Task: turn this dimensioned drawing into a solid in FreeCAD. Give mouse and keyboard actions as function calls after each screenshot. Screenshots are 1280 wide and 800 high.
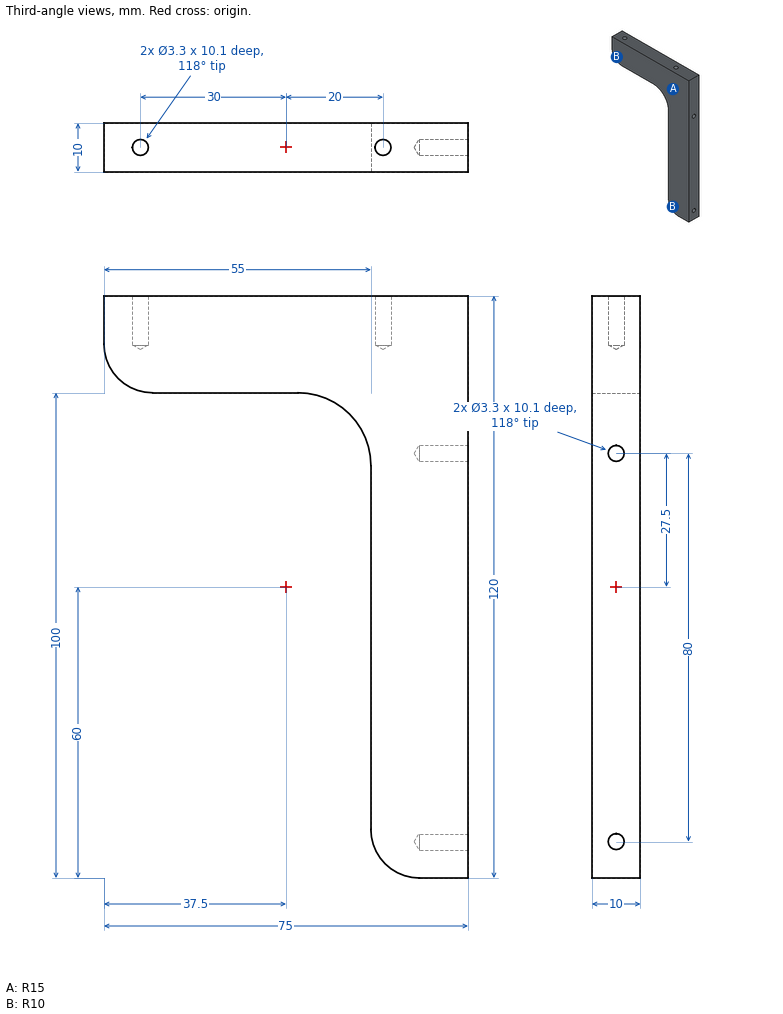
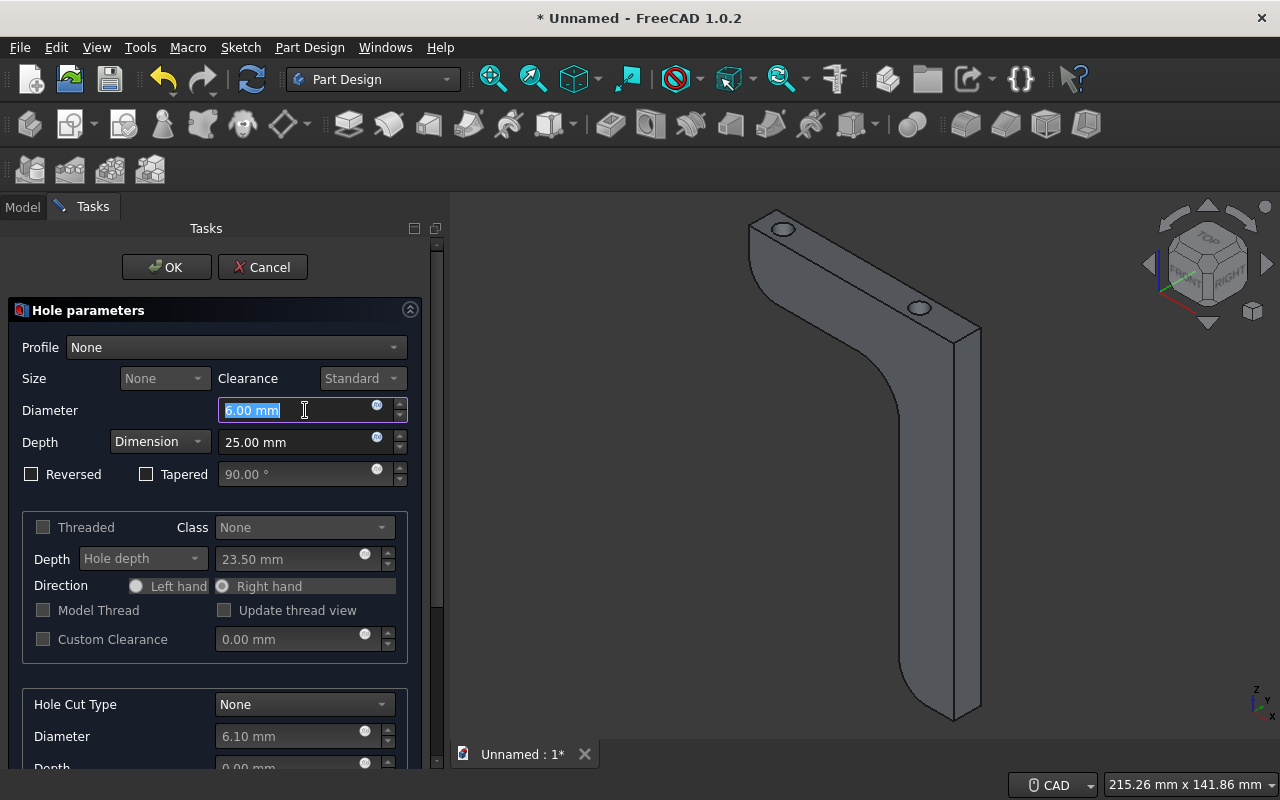
text(3.3)
key(Tab)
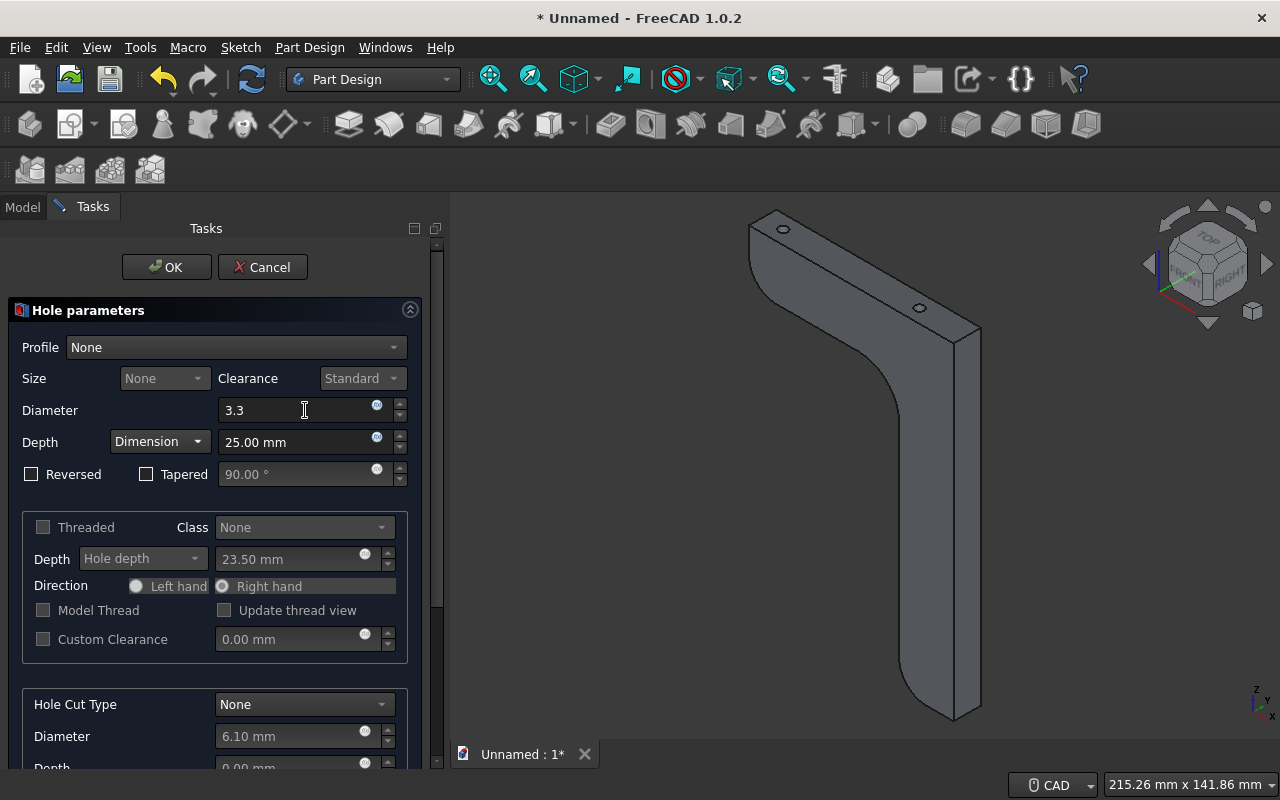
triple_click(305, 442)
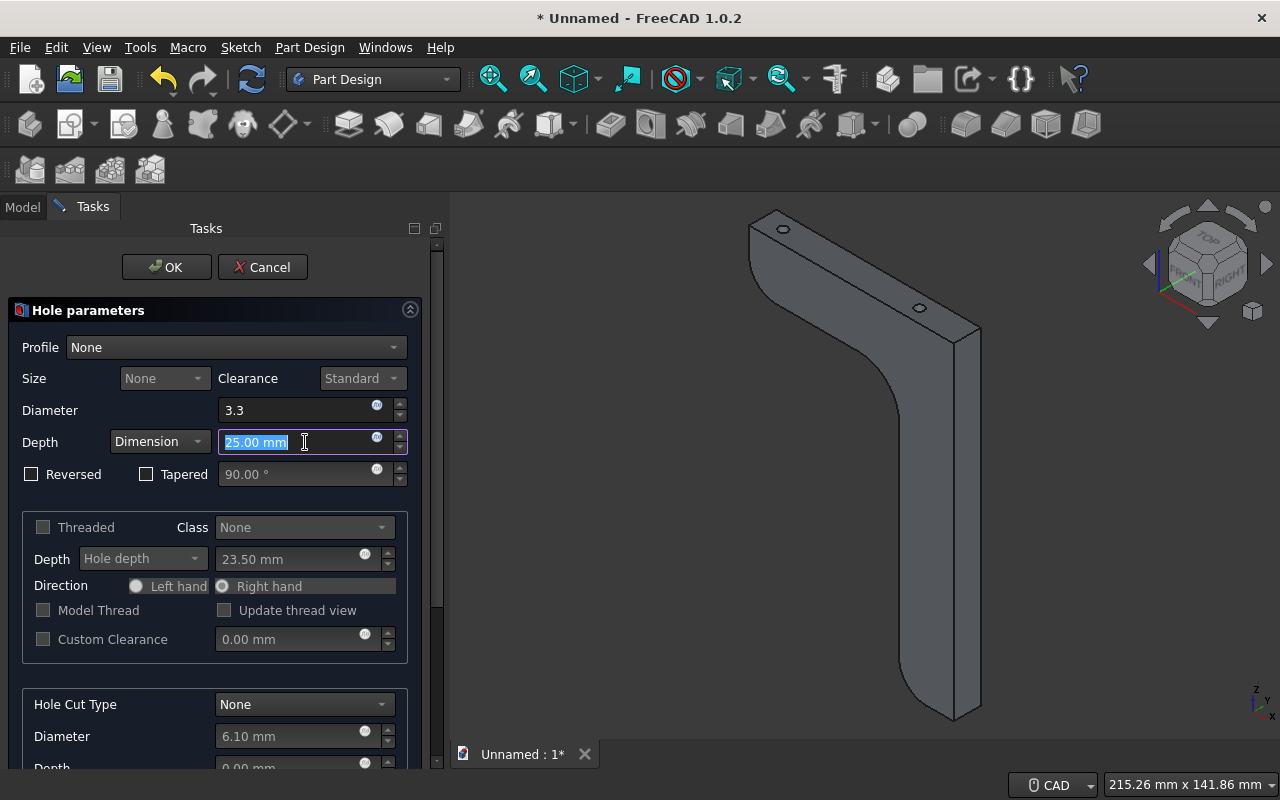
text(10.1)
key(Tab)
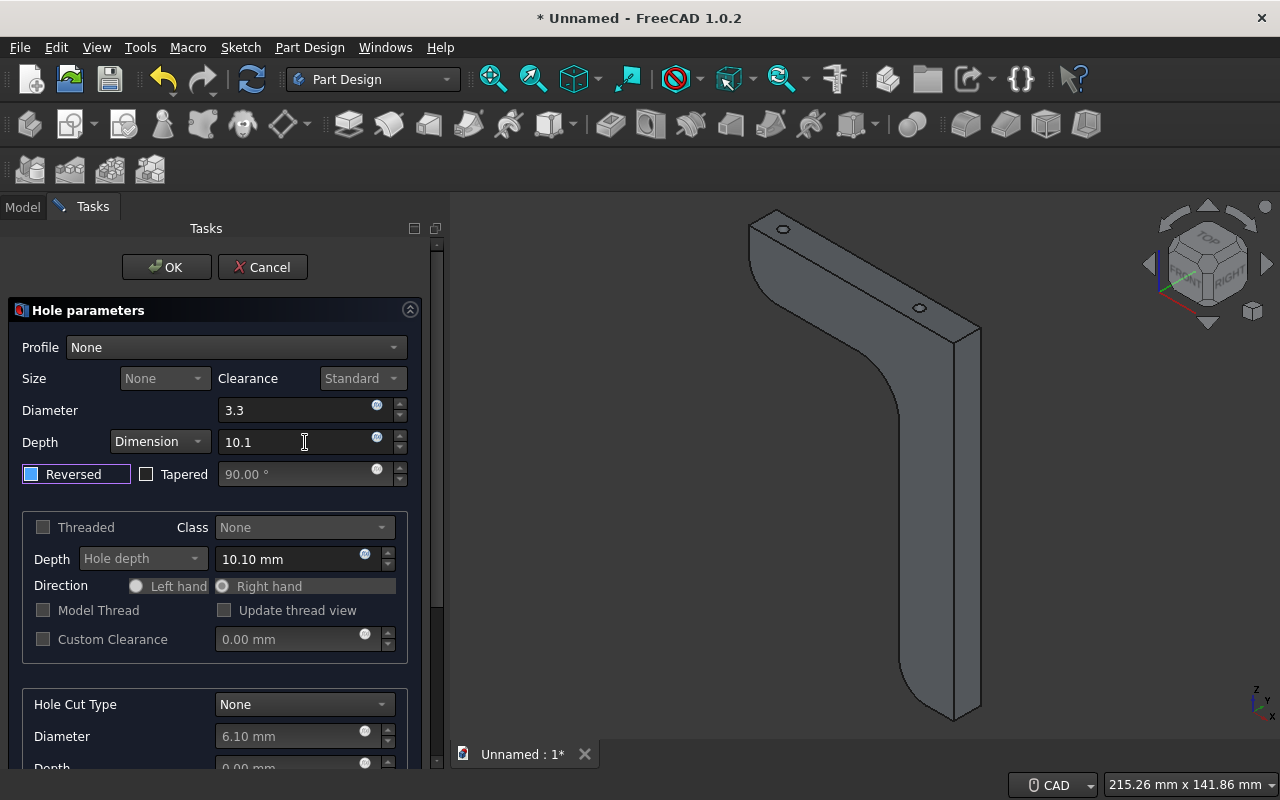
click(167, 267)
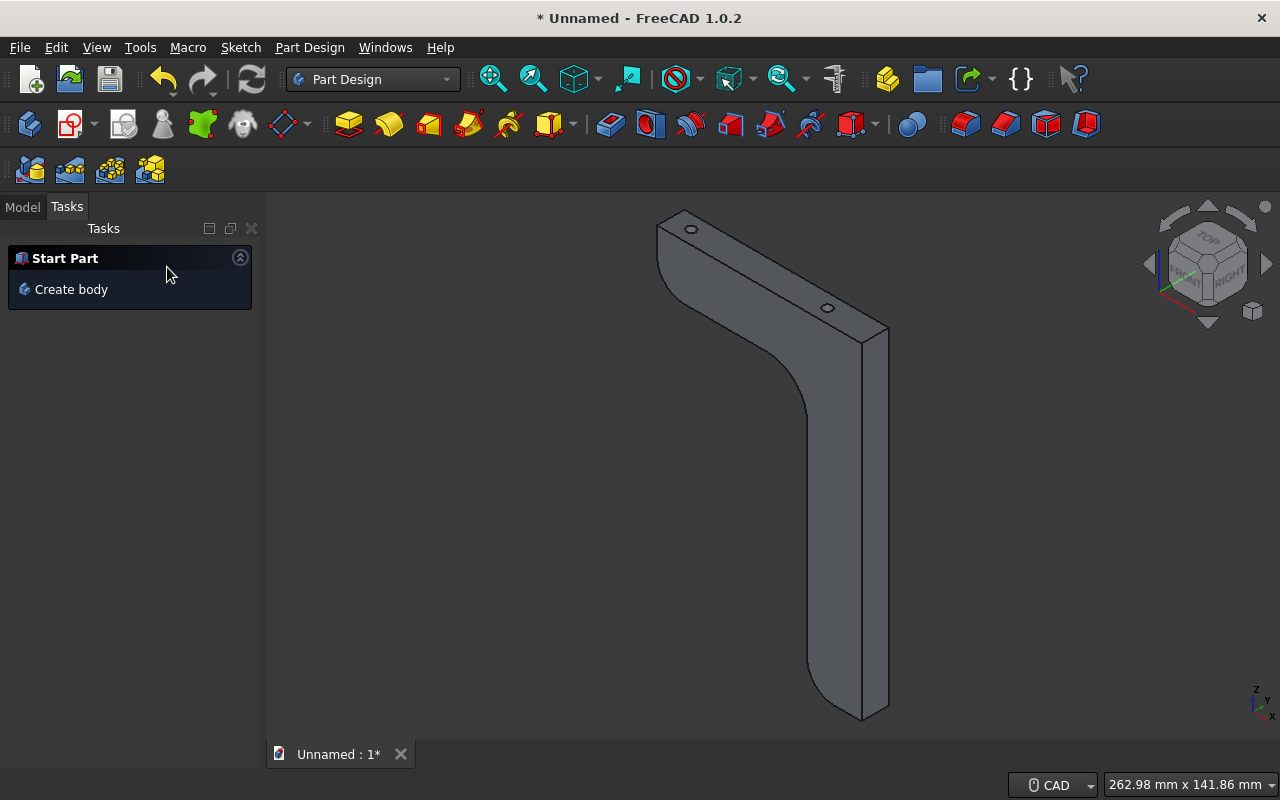
click(875, 362)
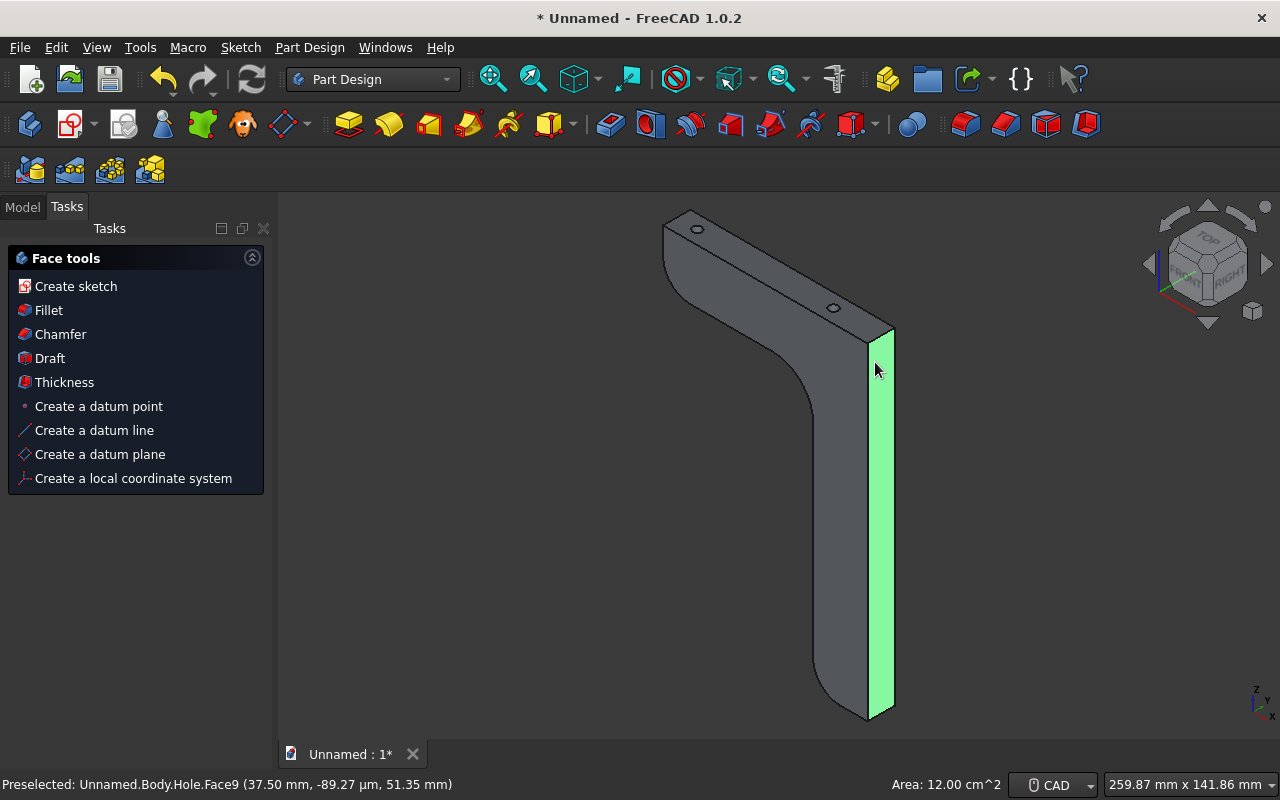
click(70, 124)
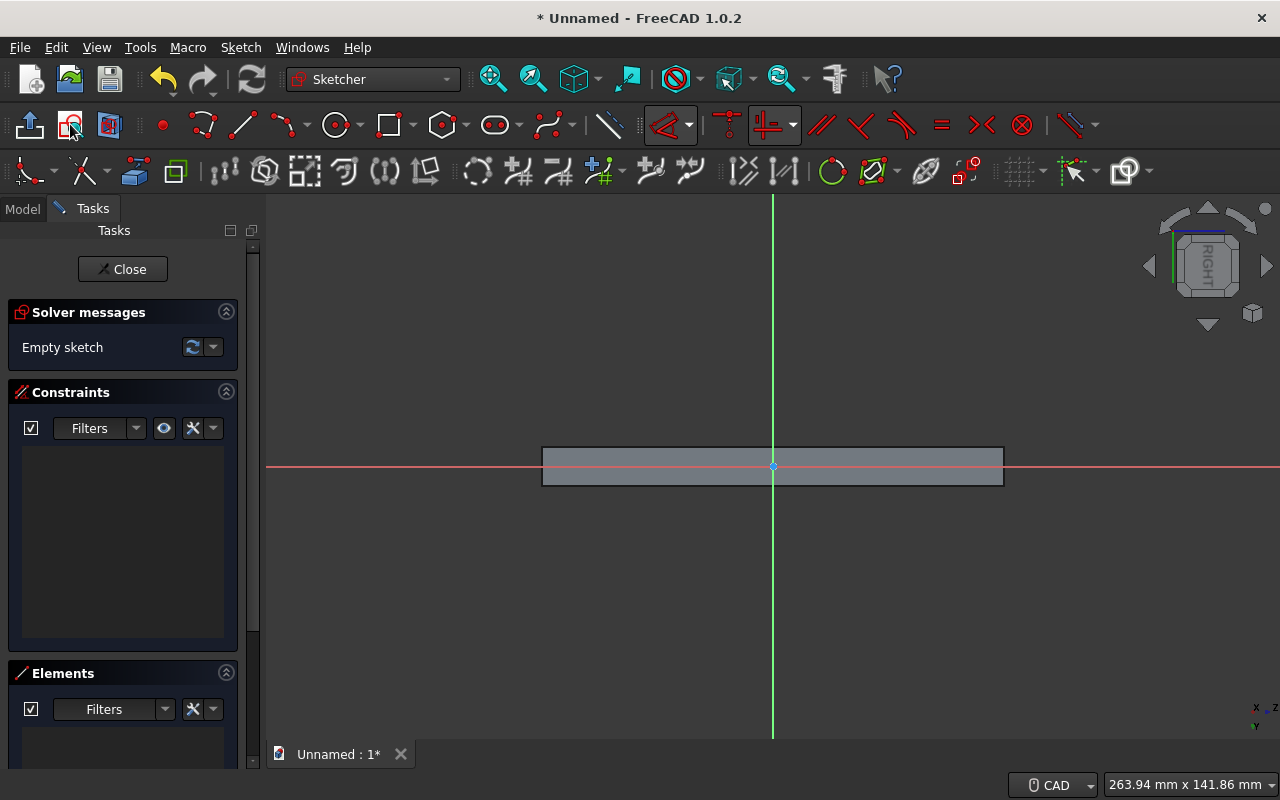
scroll(750, 467, up, 3)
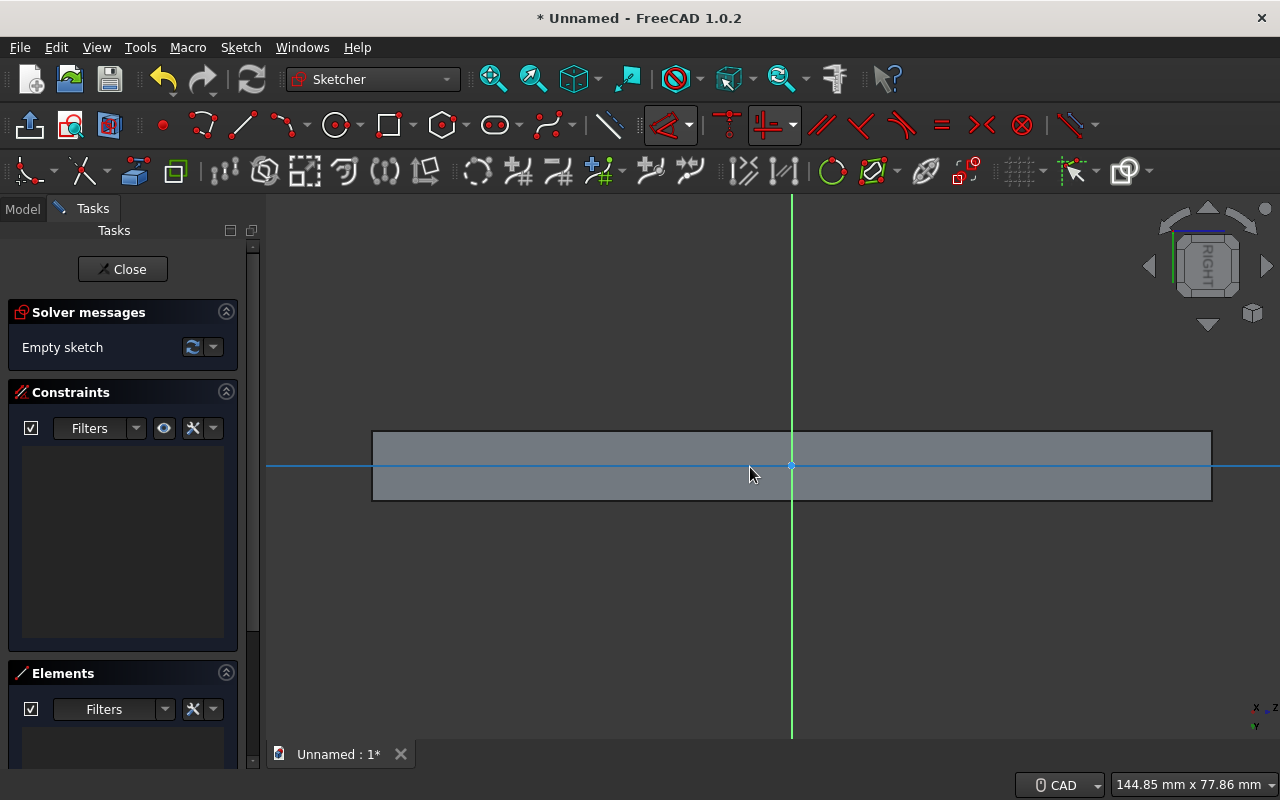
key(g)
key(c)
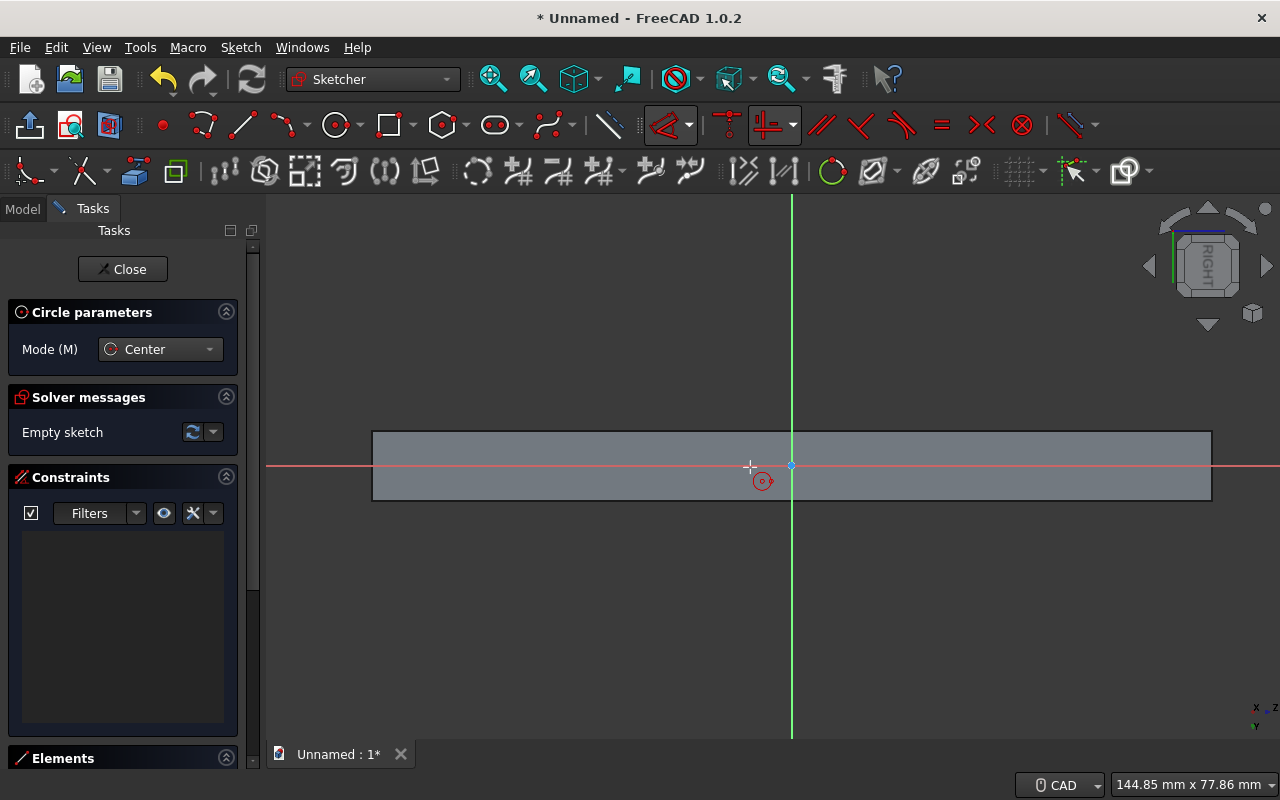
scroll(984, 466, up, 4)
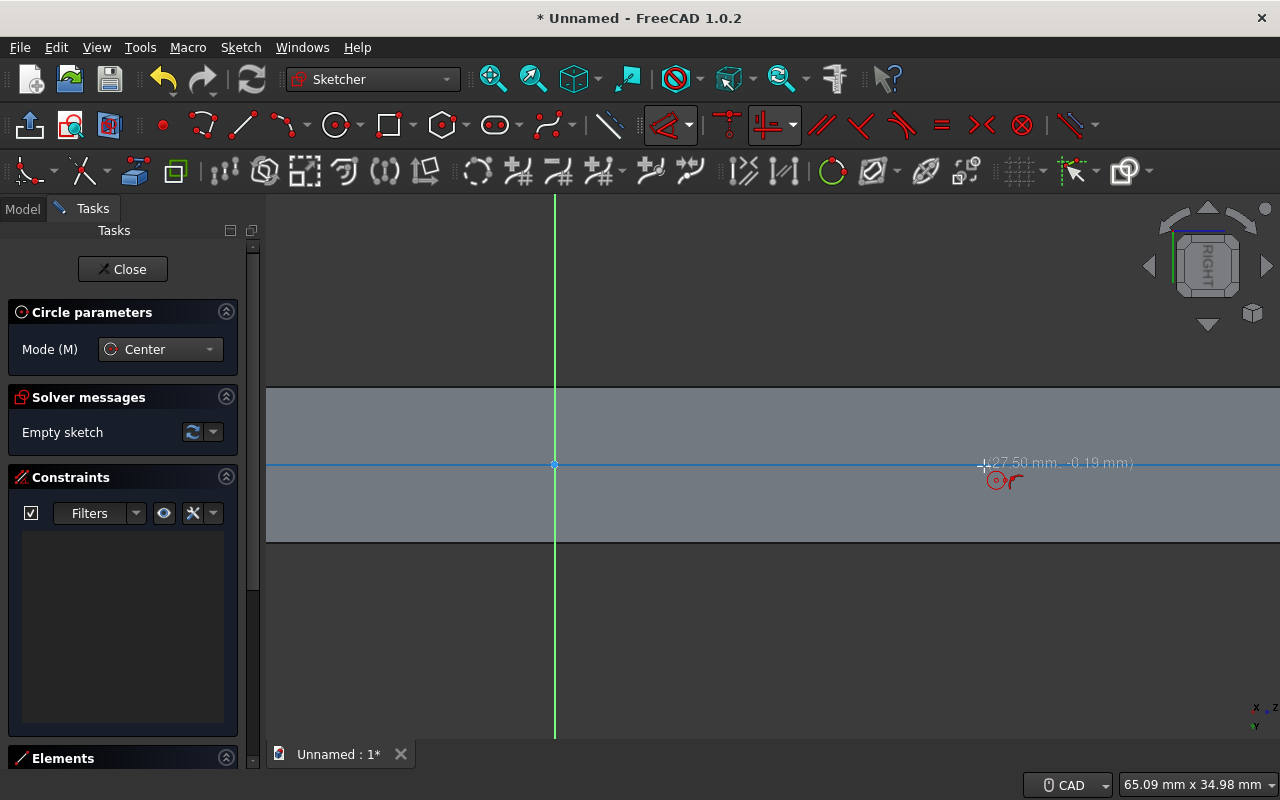
click(983, 465)
click(1001, 446)